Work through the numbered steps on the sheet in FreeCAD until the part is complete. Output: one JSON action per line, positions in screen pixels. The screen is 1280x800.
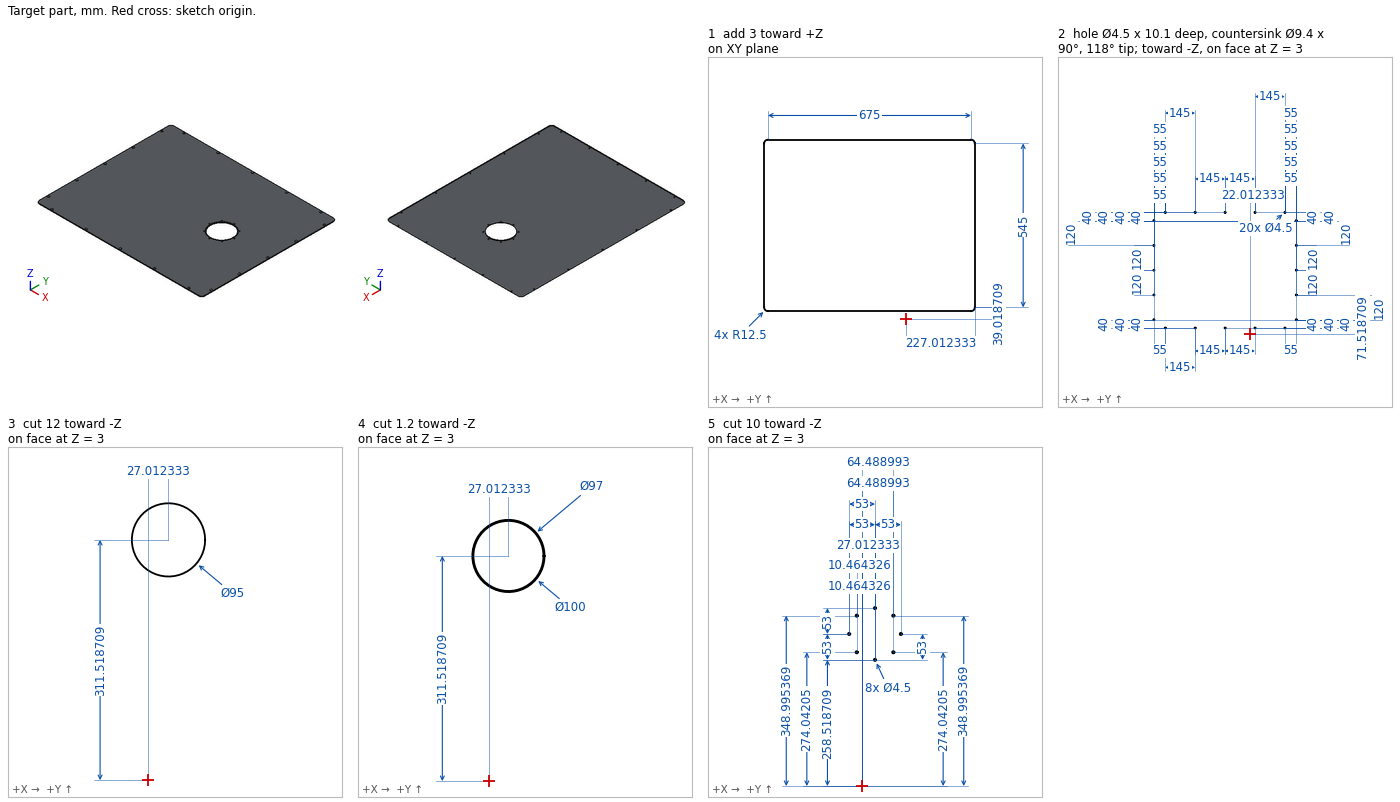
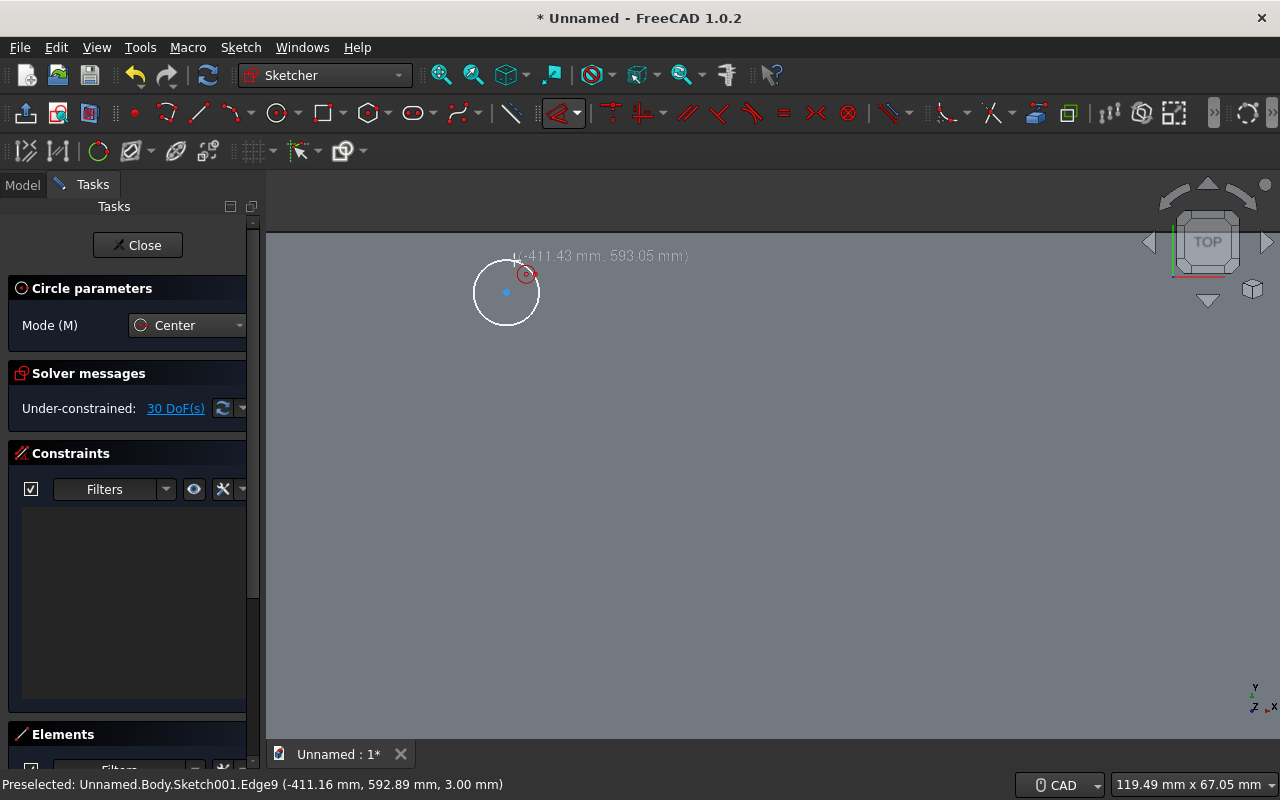
{"action": "scroll", "coordinate": [523, 268], "scroll_direction": "down", "scroll_amount": 13}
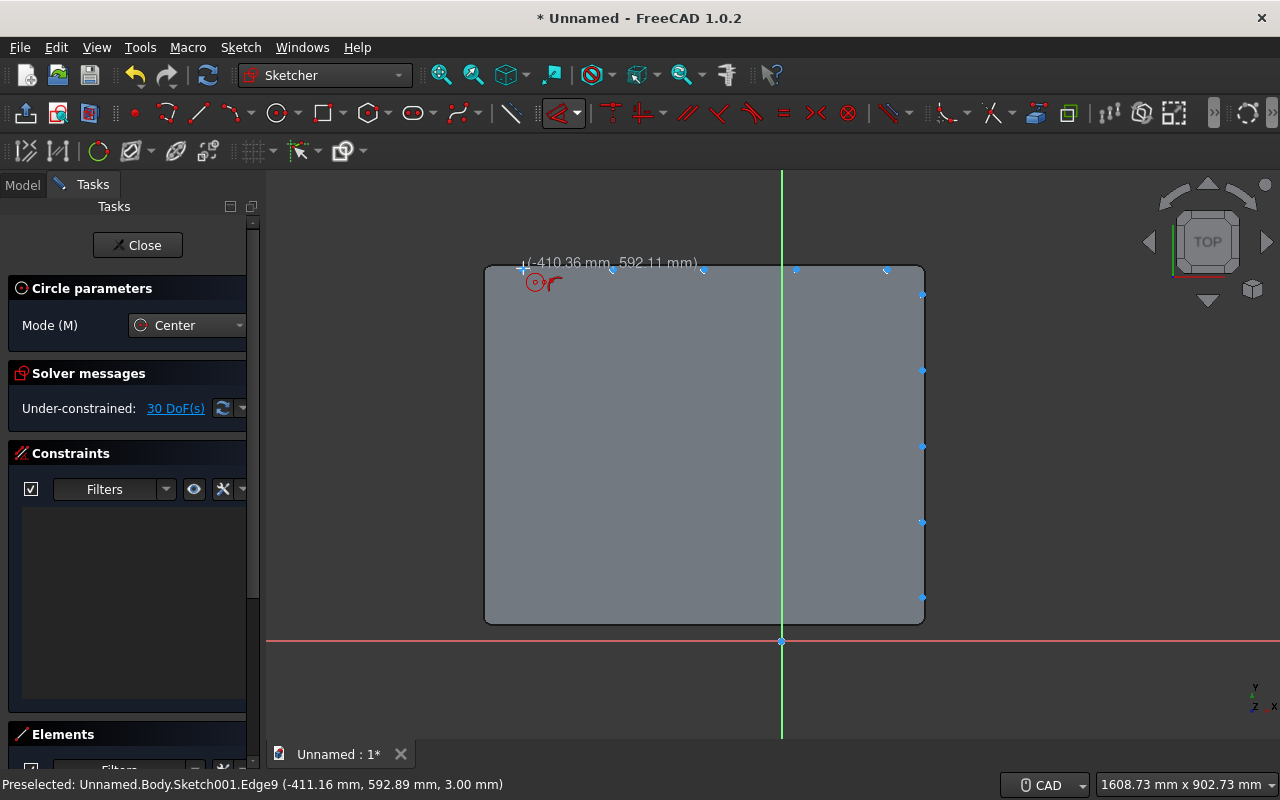
{"action": "scroll", "coordinate": [487, 294], "scroll_direction": "up", "scroll_amount": 14}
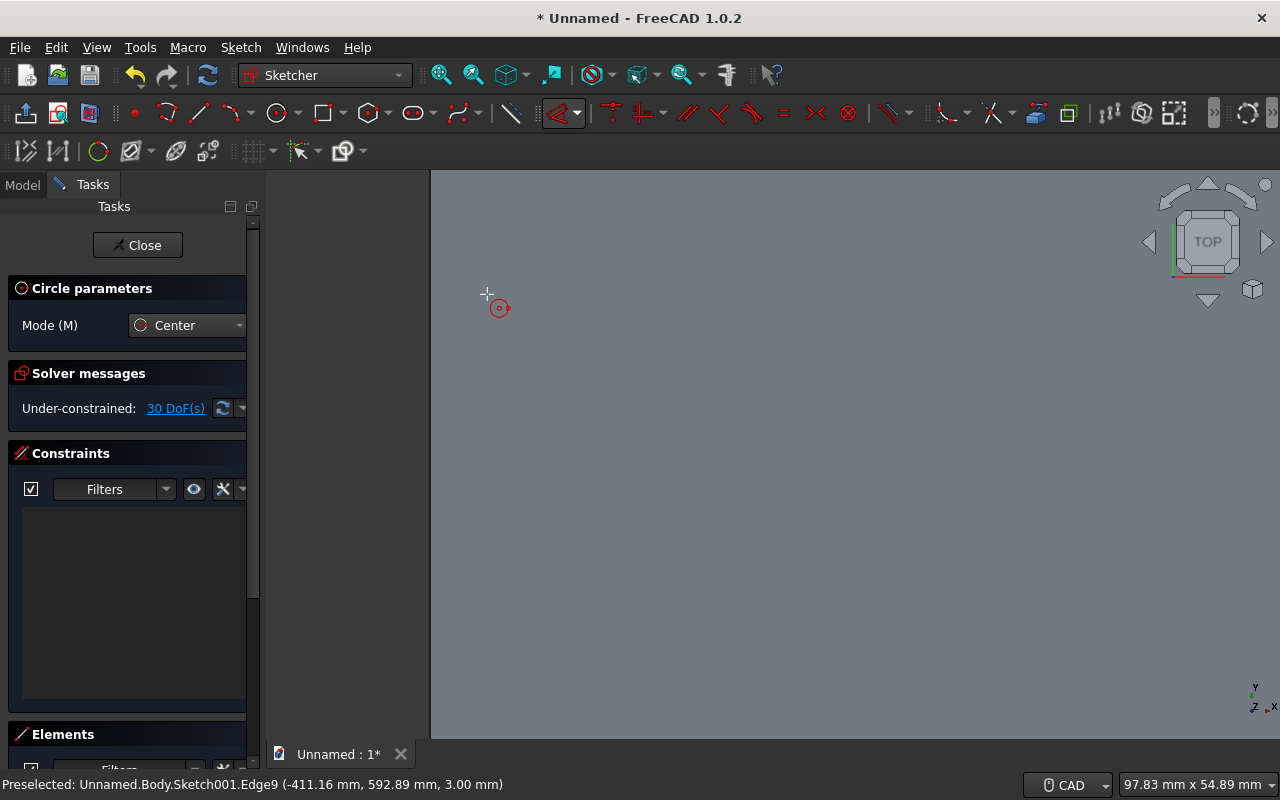
{"action": "scroll", "coordinate": [487, 294], "scroll_direction": "down", "scroll_amount": 14}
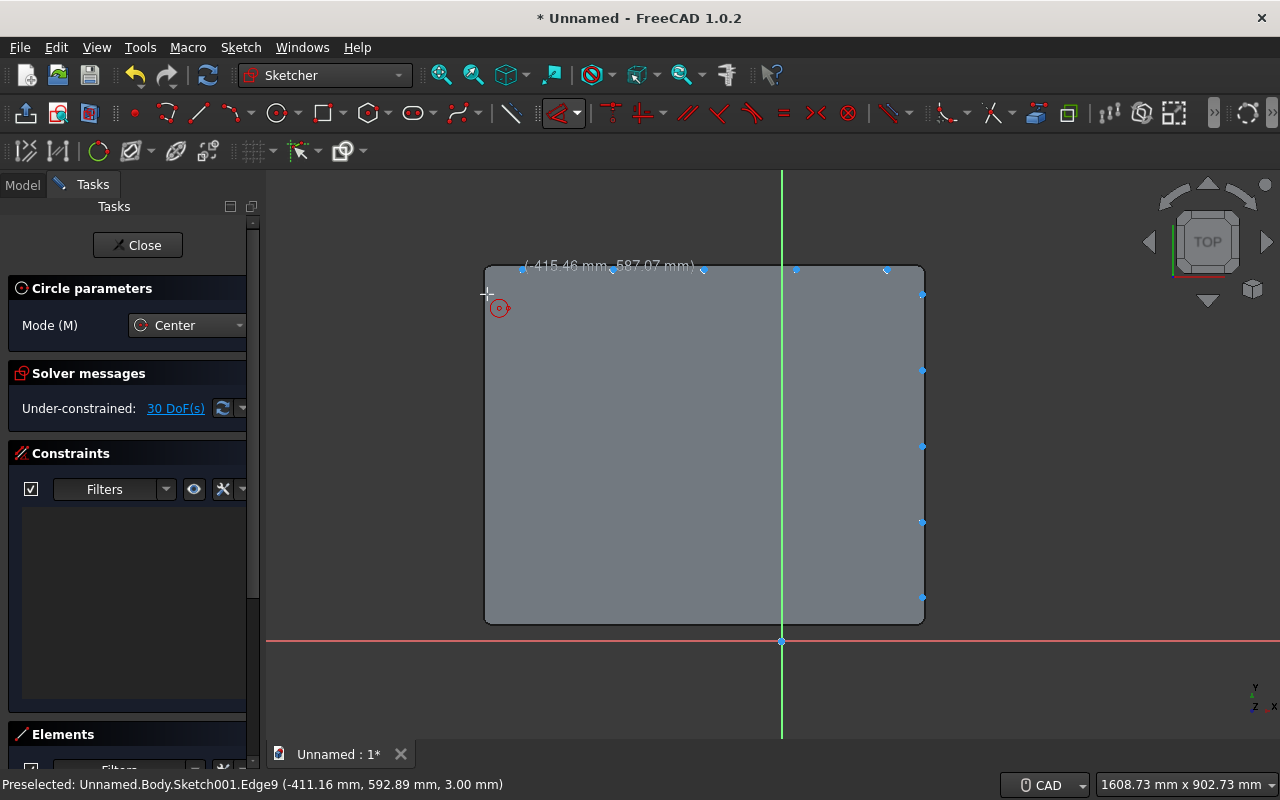
{"action": "left_click", "coordinate": [487, 294]}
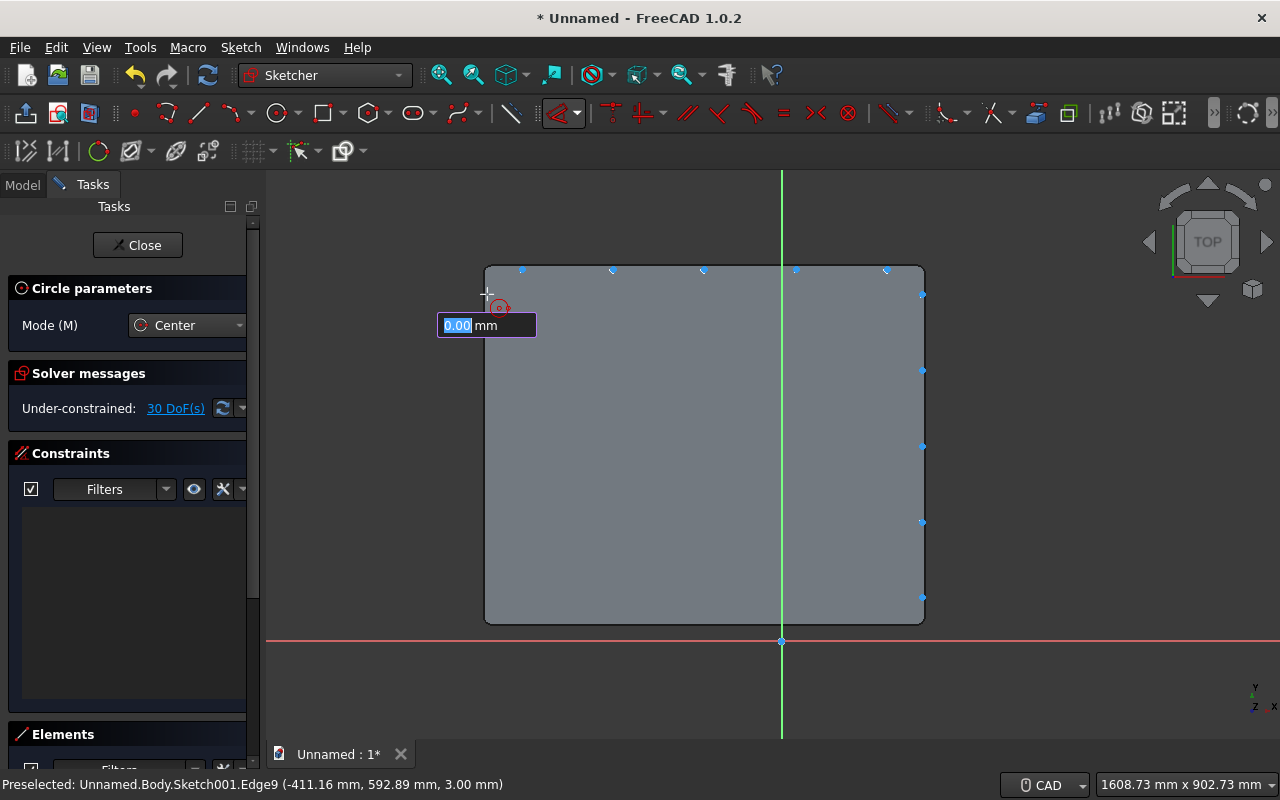
{"action": "scroll", "coordinate": [488, 293], "scroll_direction": "up", "scroll_amount": 13}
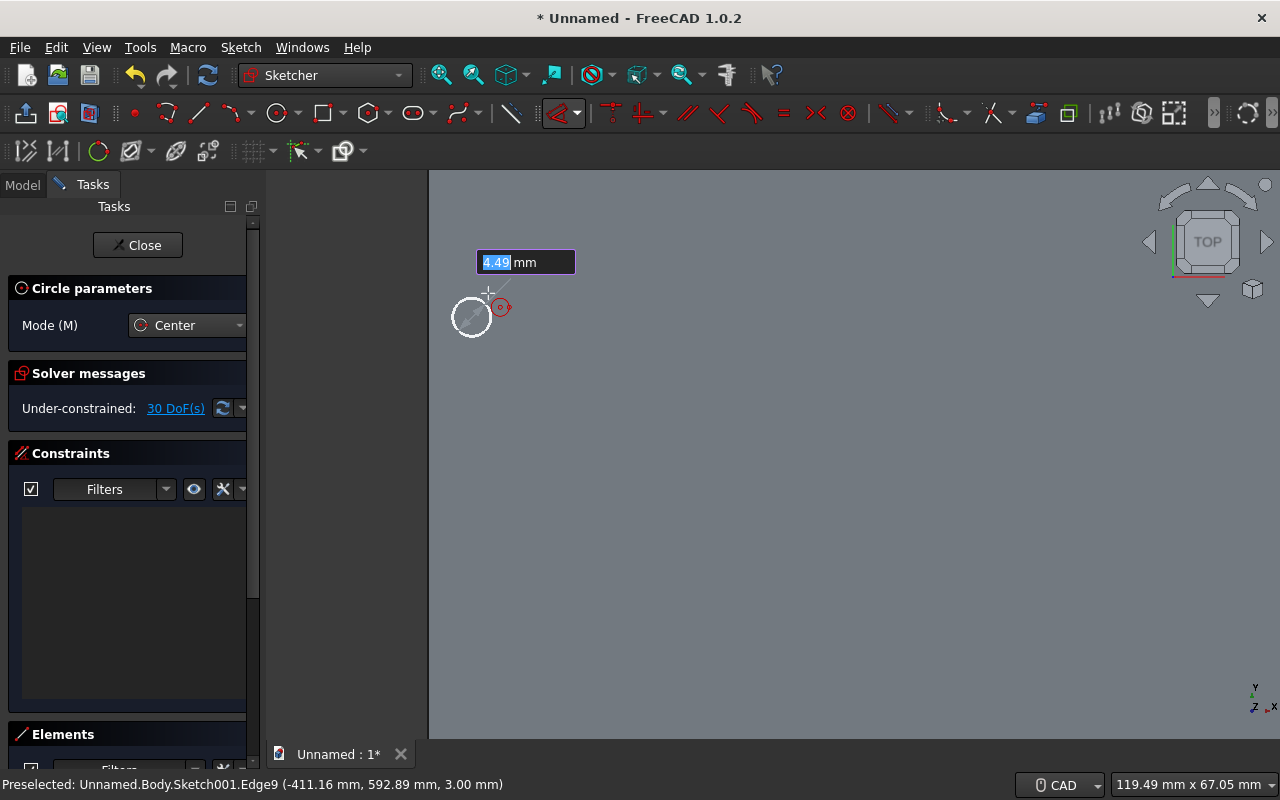
{"action": "left_click", "coordinate": [484, 288]}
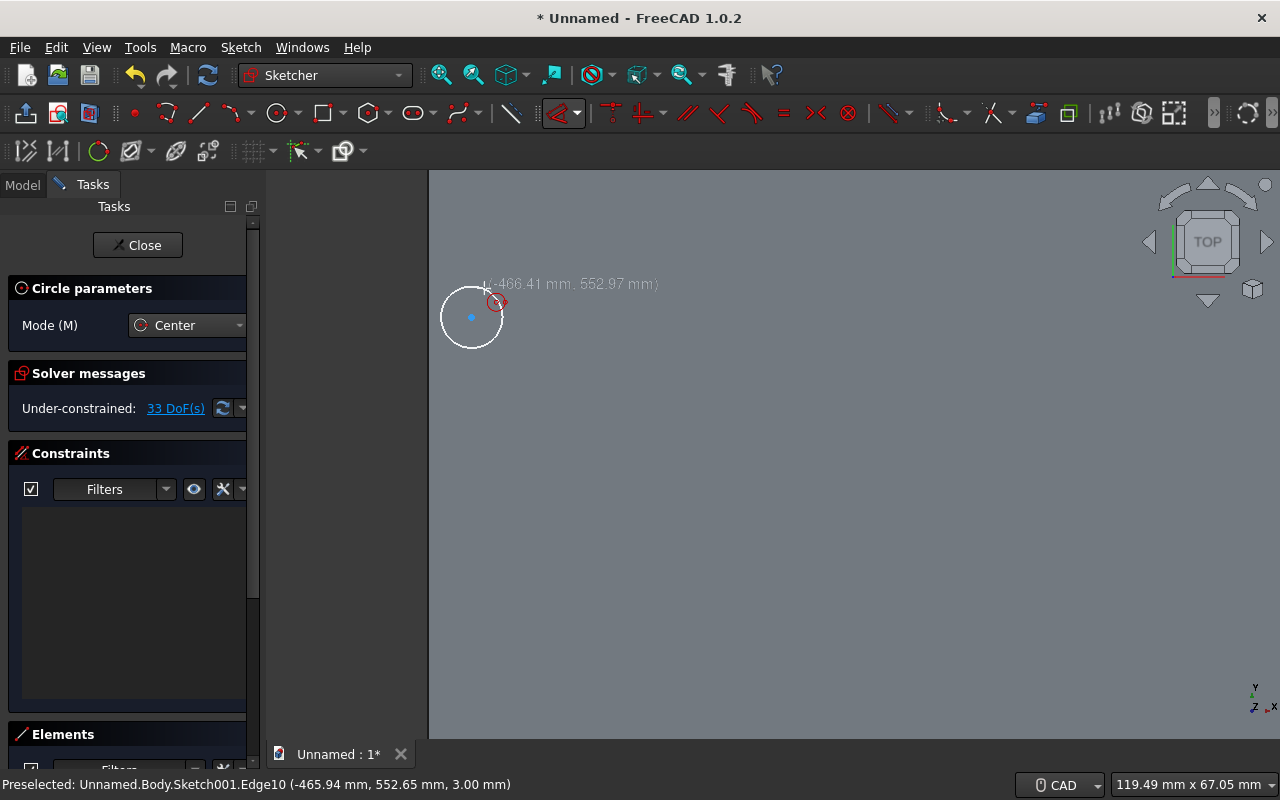
{"action": "scroll", "coordinate": [488, 293], "scroll_direction": "down", "scroll_amount": 13}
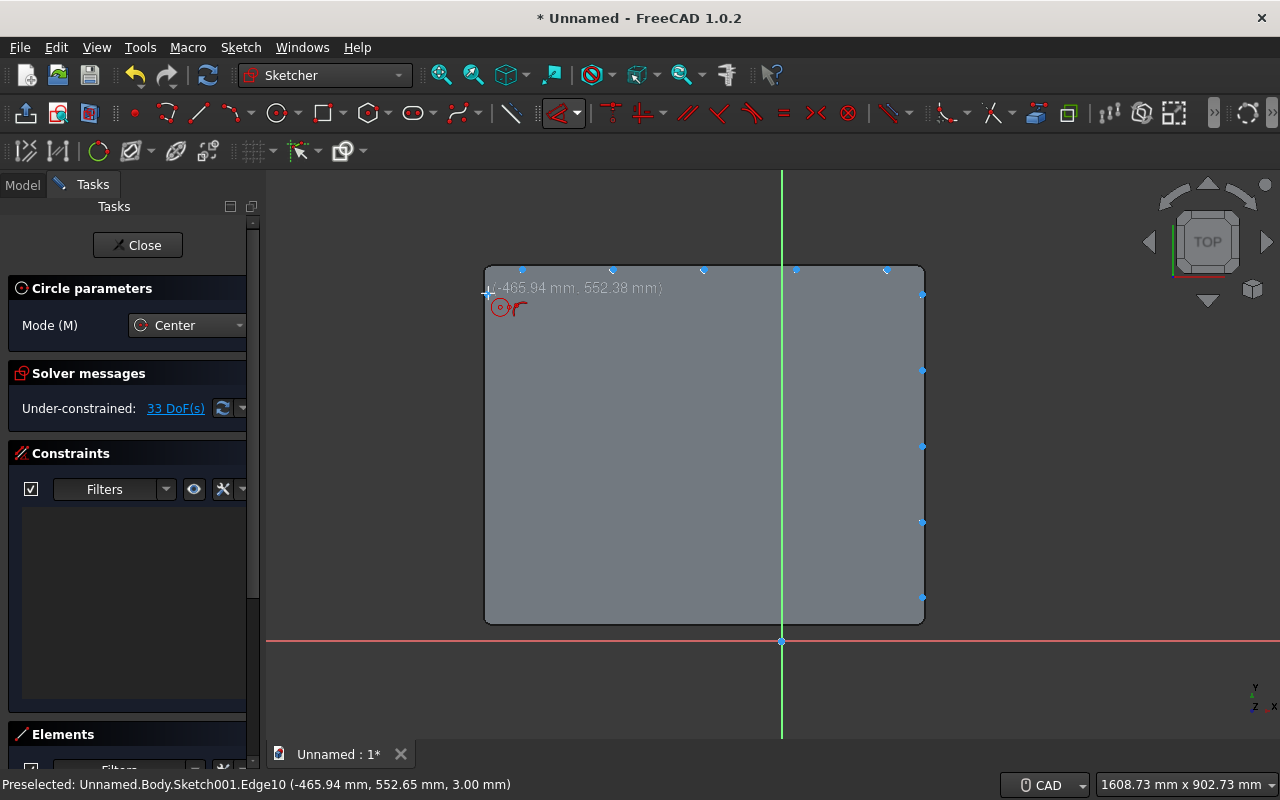
{"action": "scroll", "coordinate": [487, 369], "scroll_direction": "up", "scroll_amount": 14}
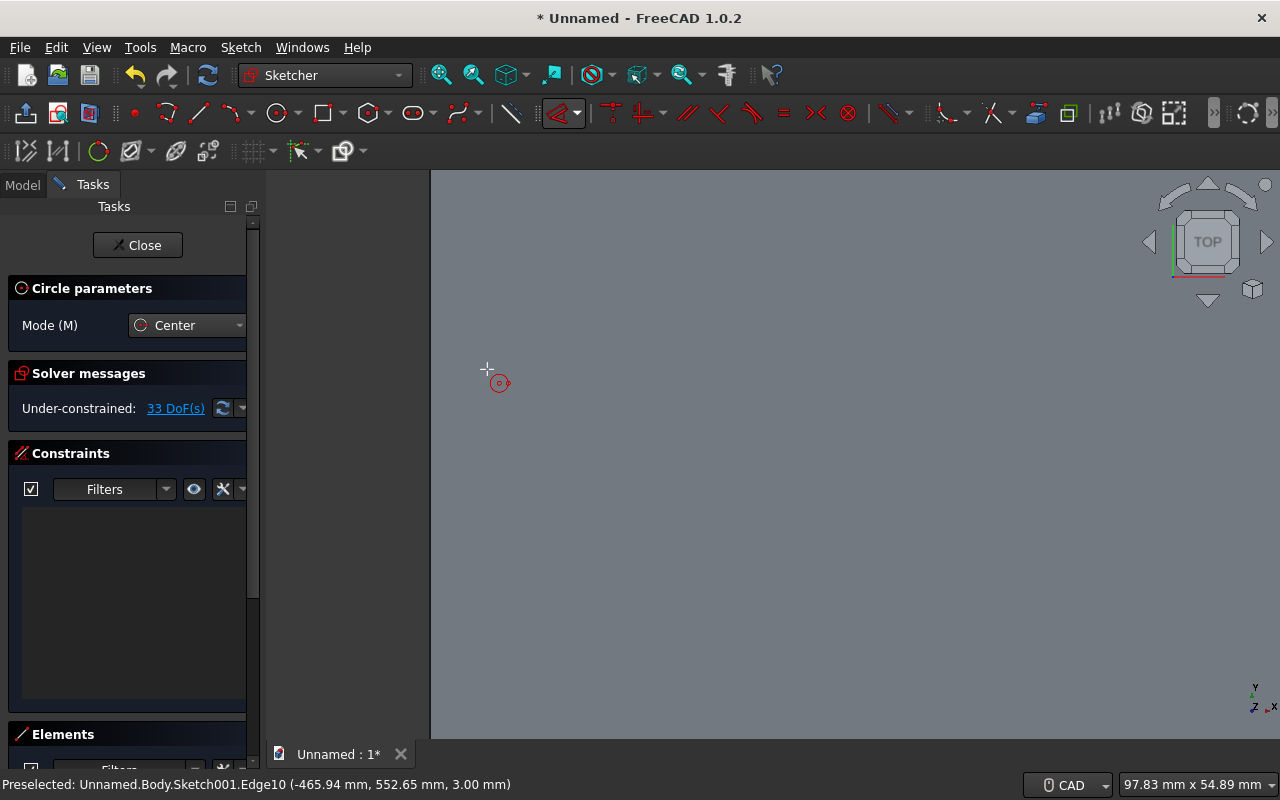
{"action": "scroll", "coordinate": [487, 370], "scroll_direction": "down", "scroll_amount": 14}